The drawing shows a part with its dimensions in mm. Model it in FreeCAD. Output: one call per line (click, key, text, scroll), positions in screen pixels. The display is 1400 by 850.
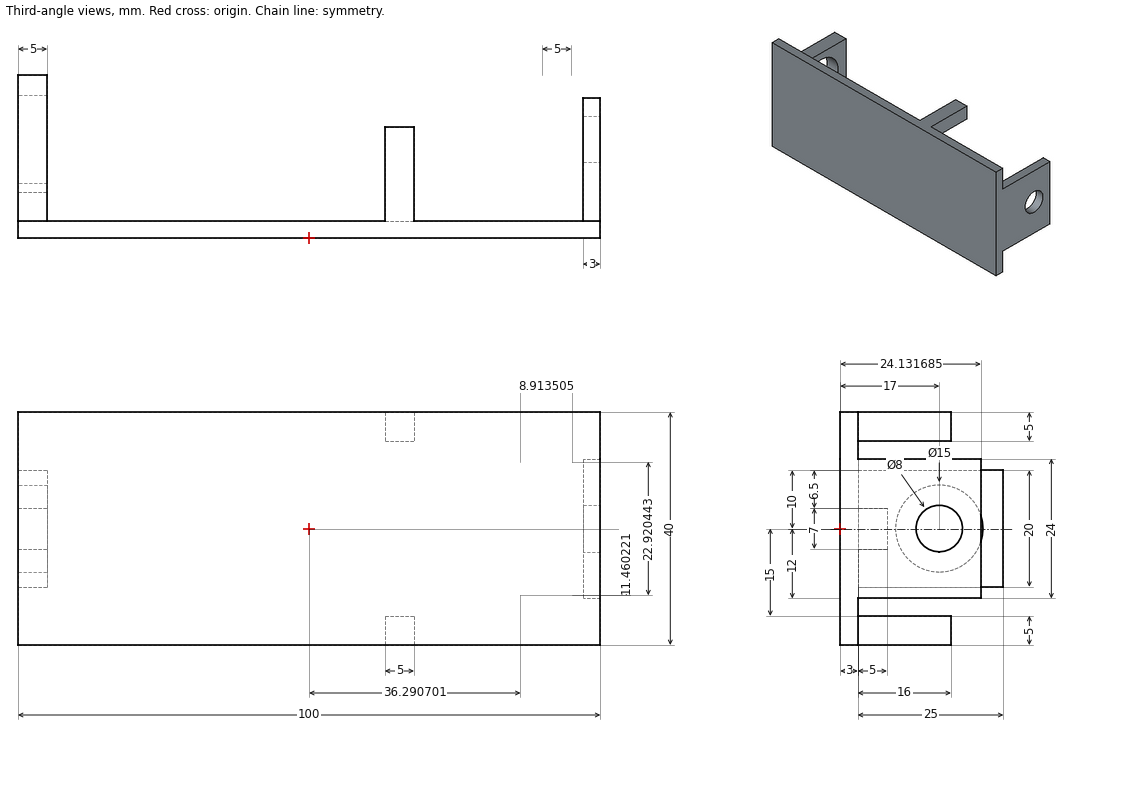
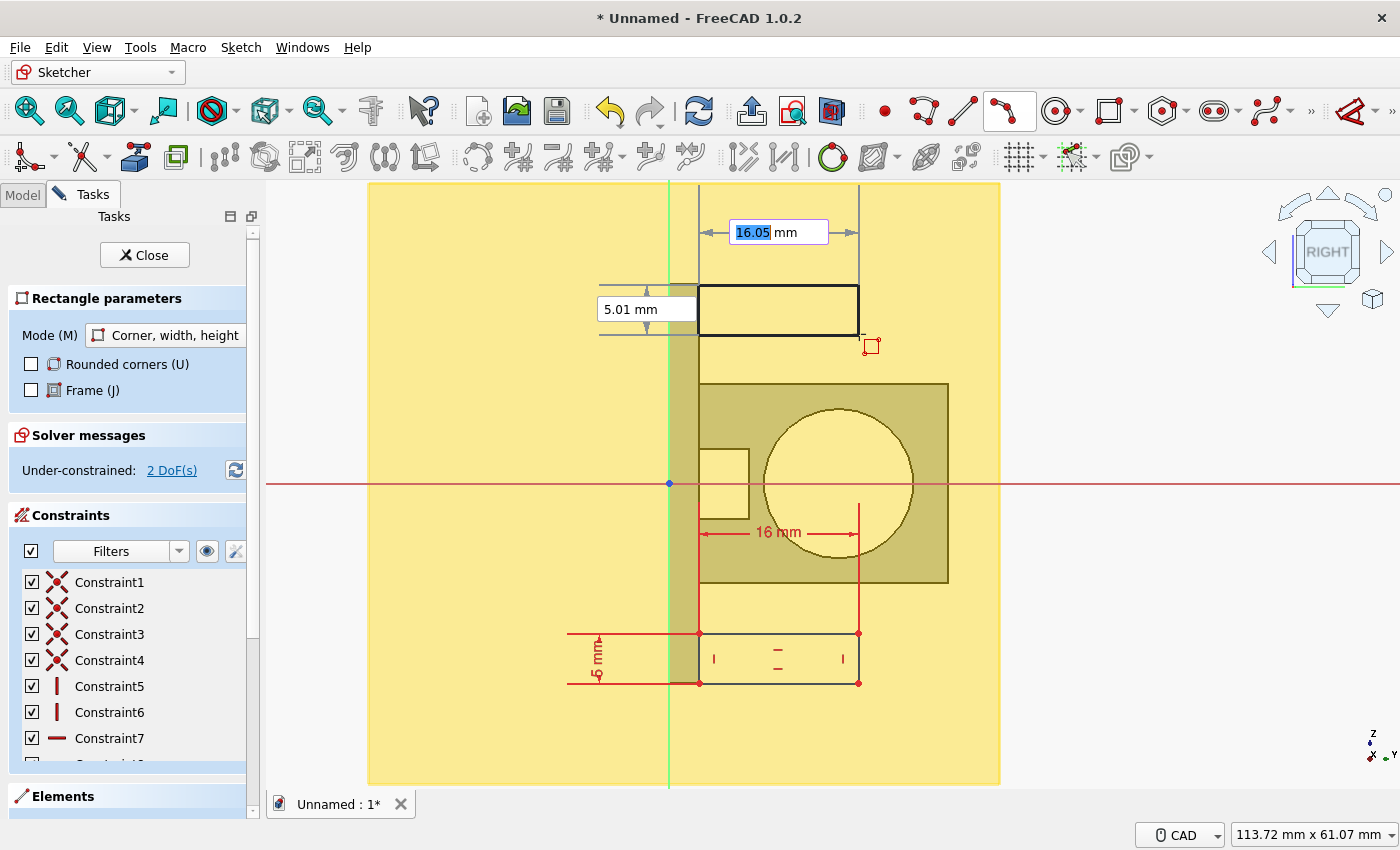
text(16)
key(Tab)
text(5)
key(Return)
key(Escape)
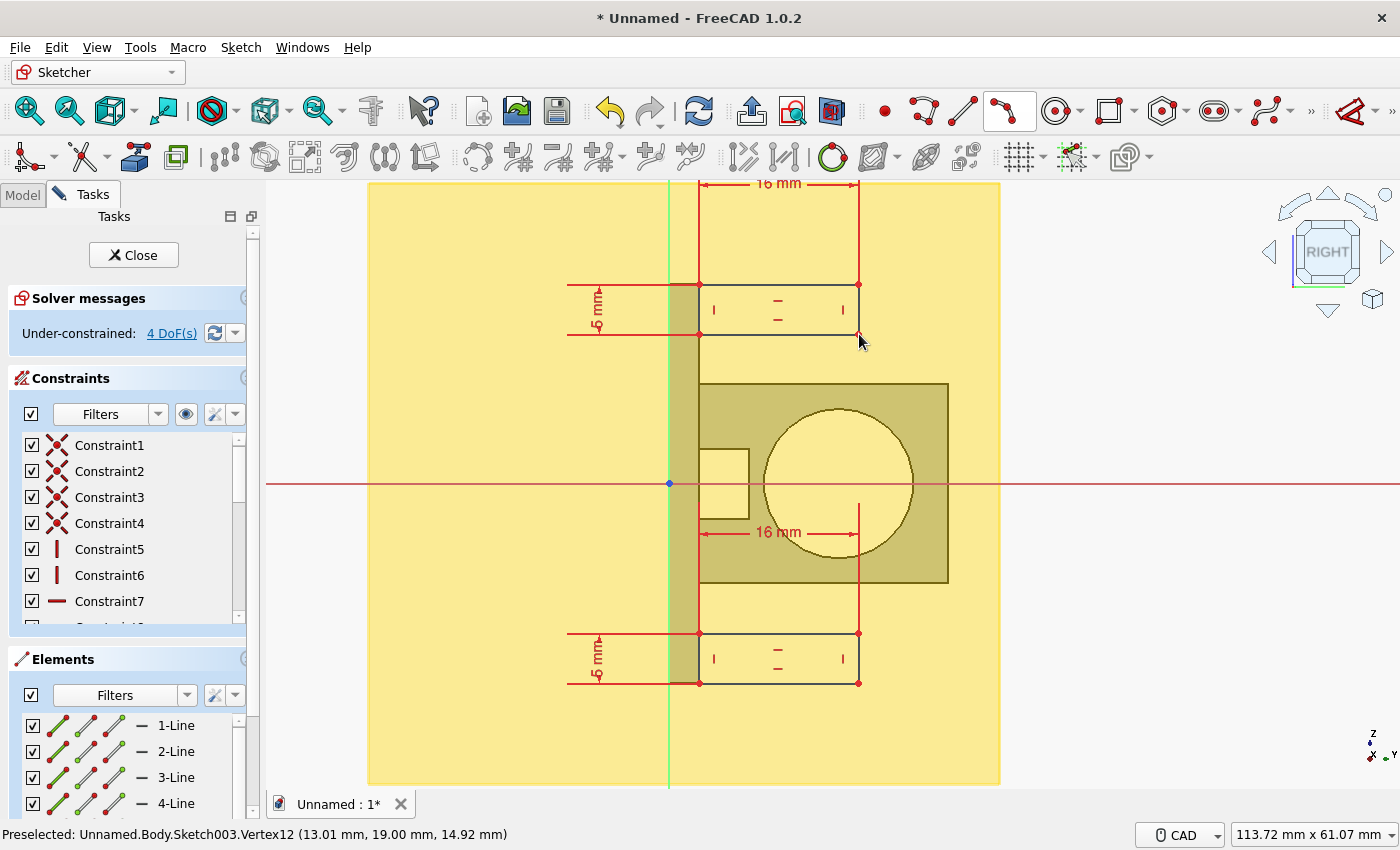
click(699, 684)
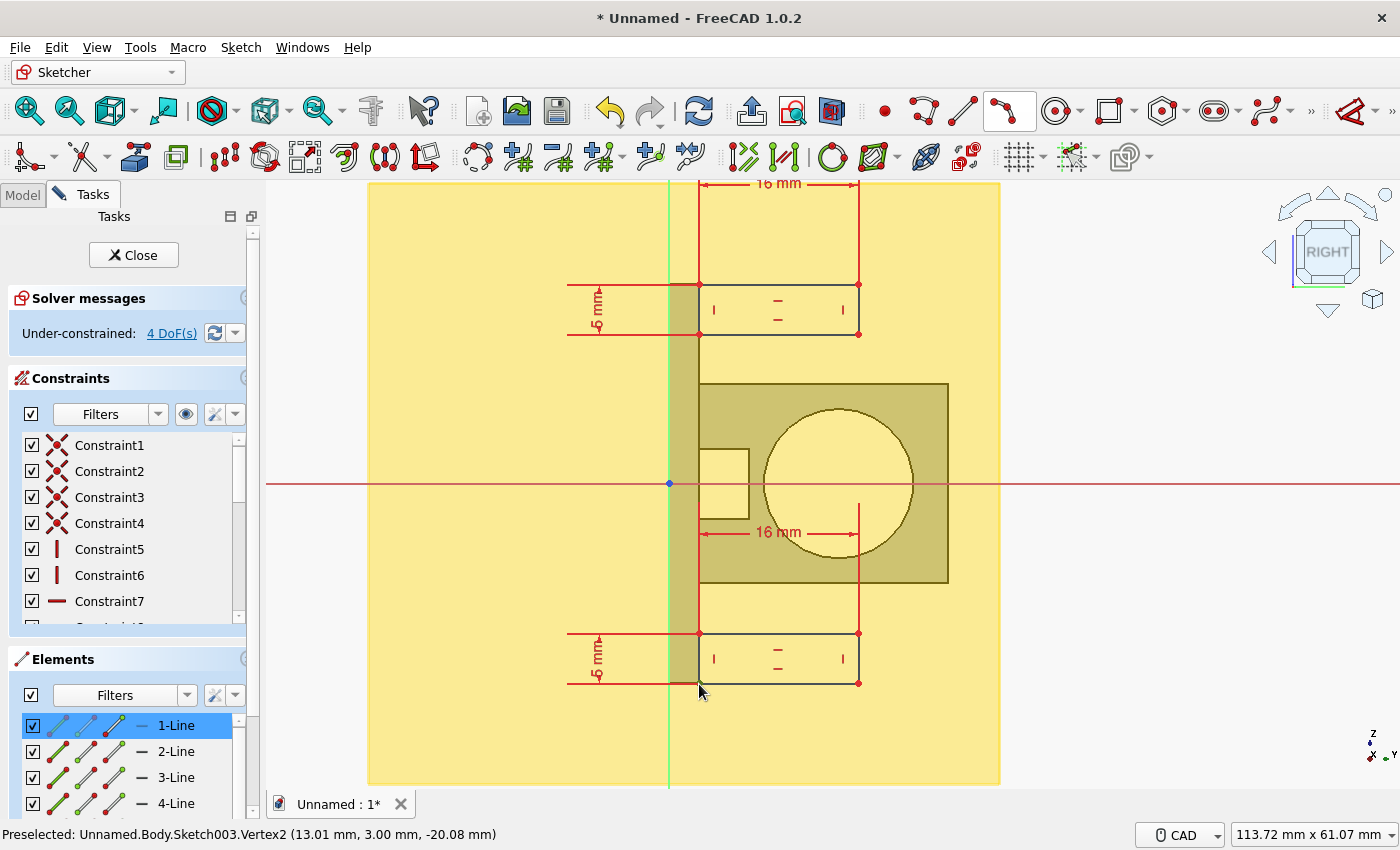
click(699, 285)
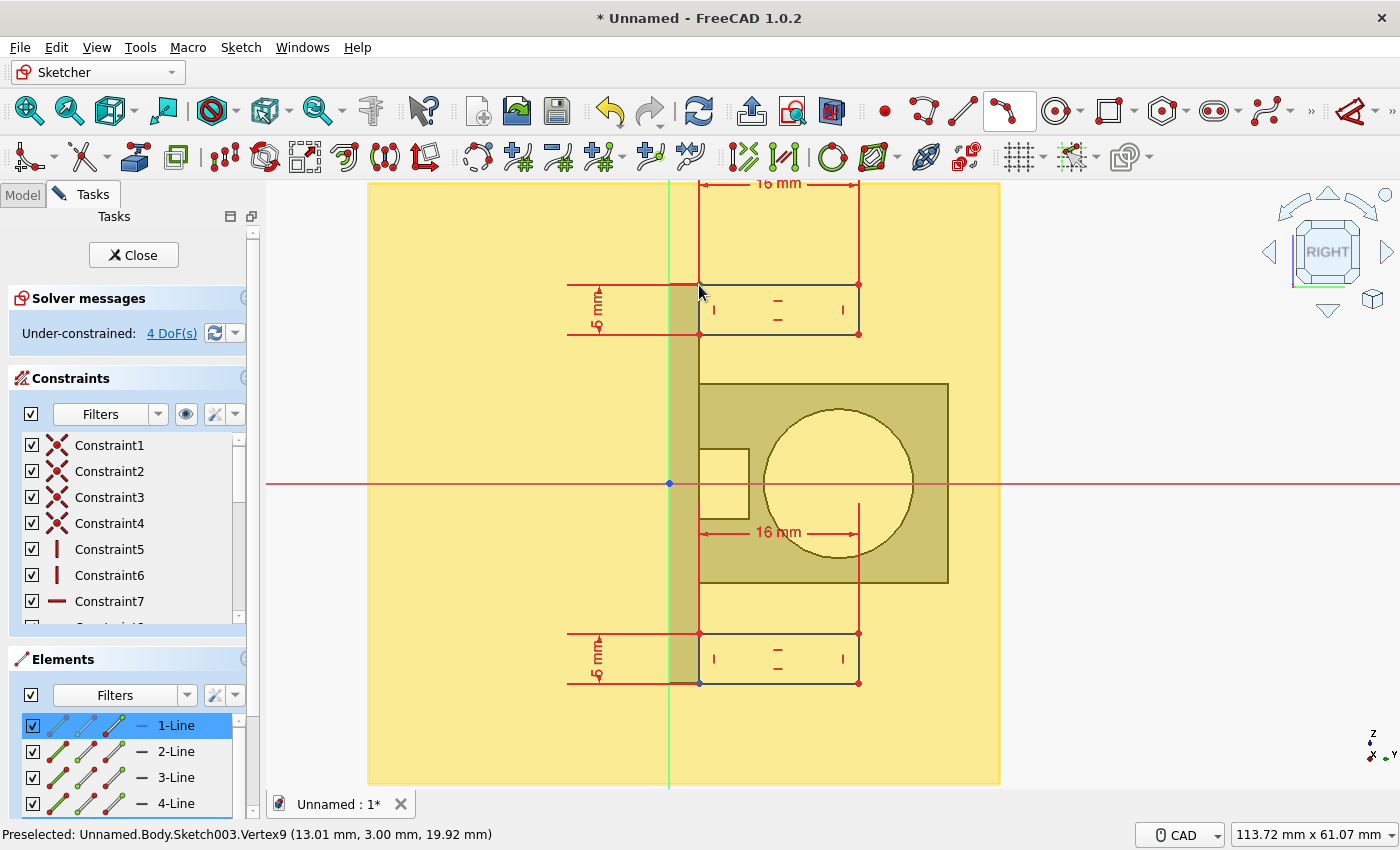
click(361, 484)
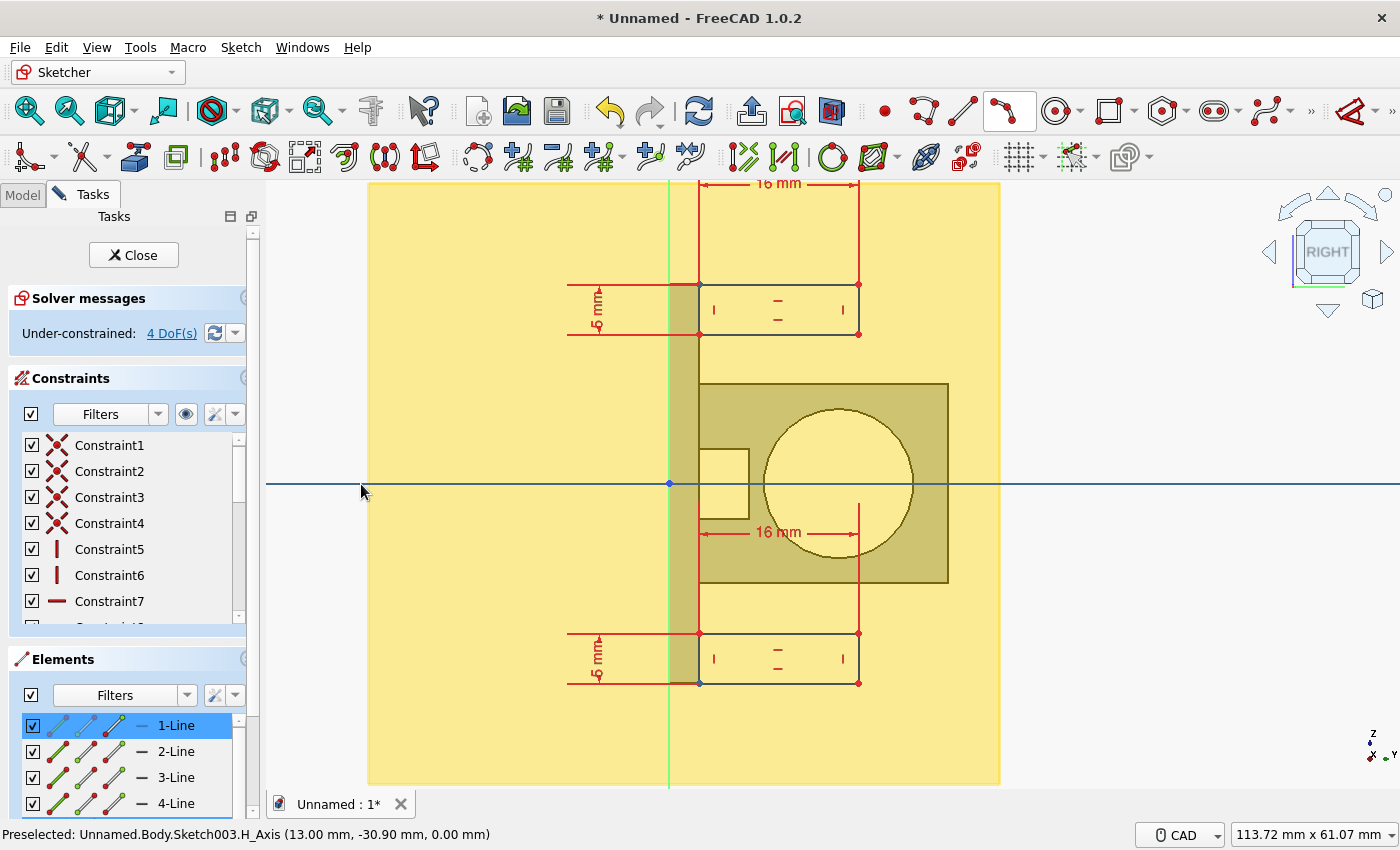
key(s)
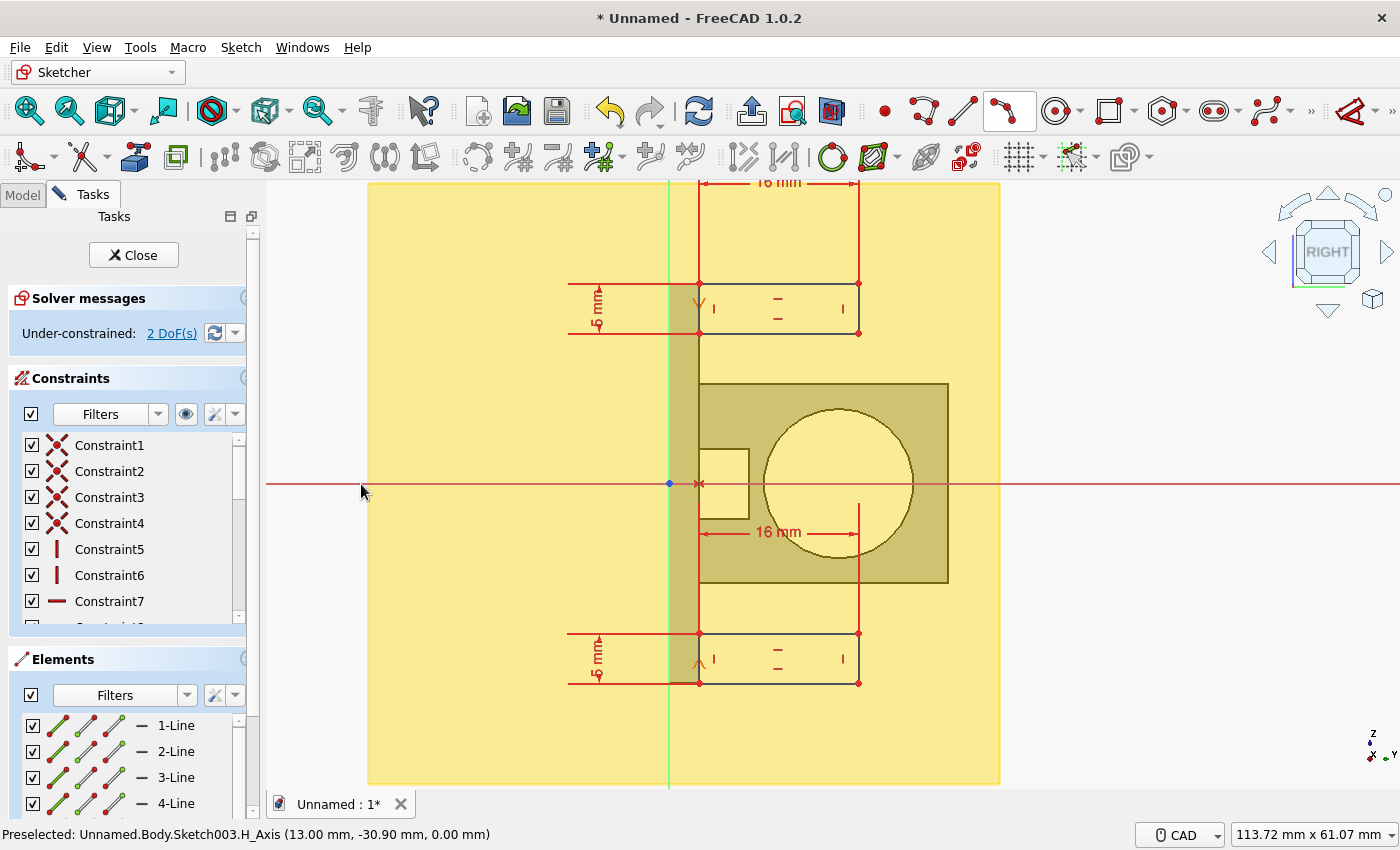
click(1350, 112)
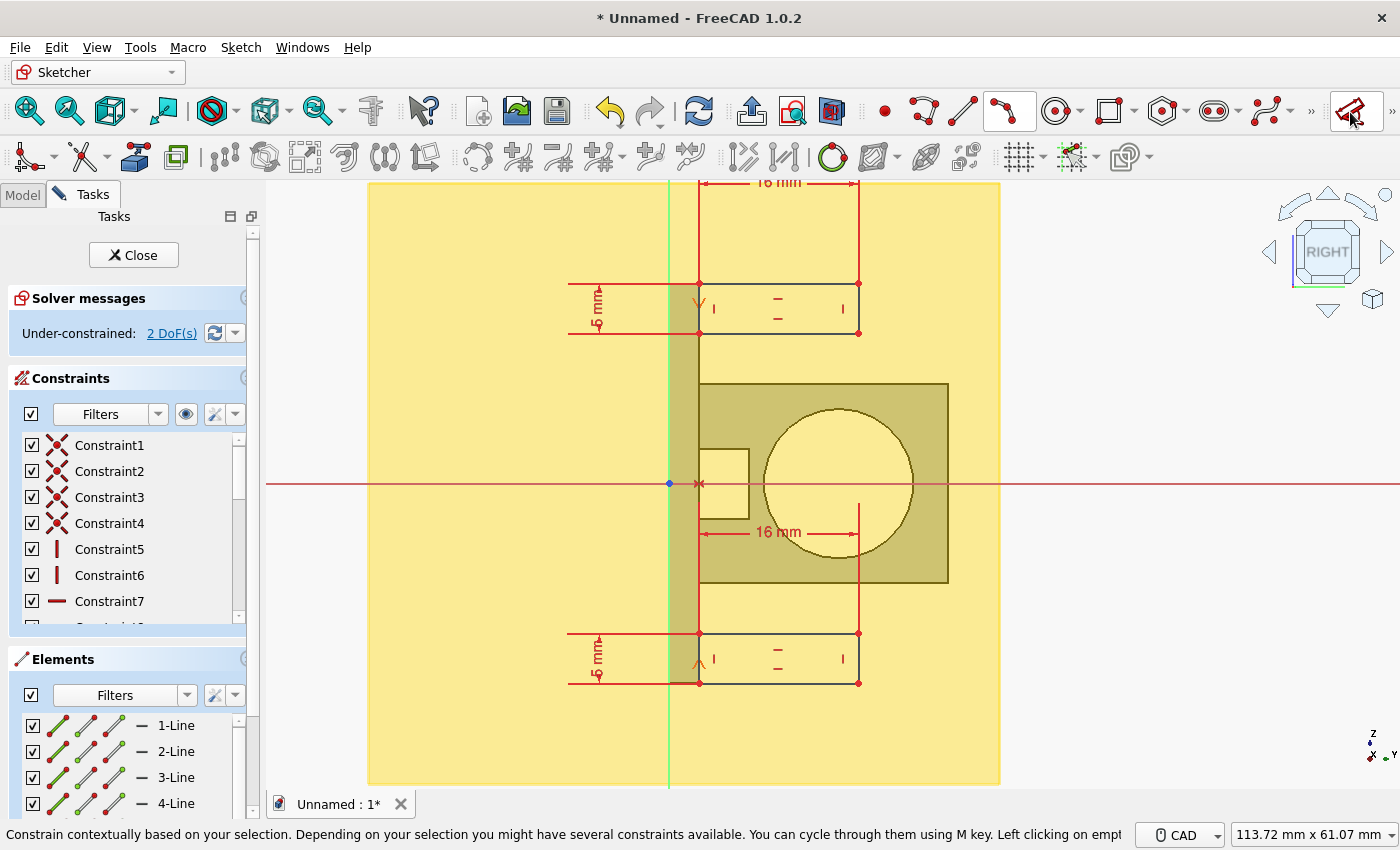
scroll(699, 634, up, 2)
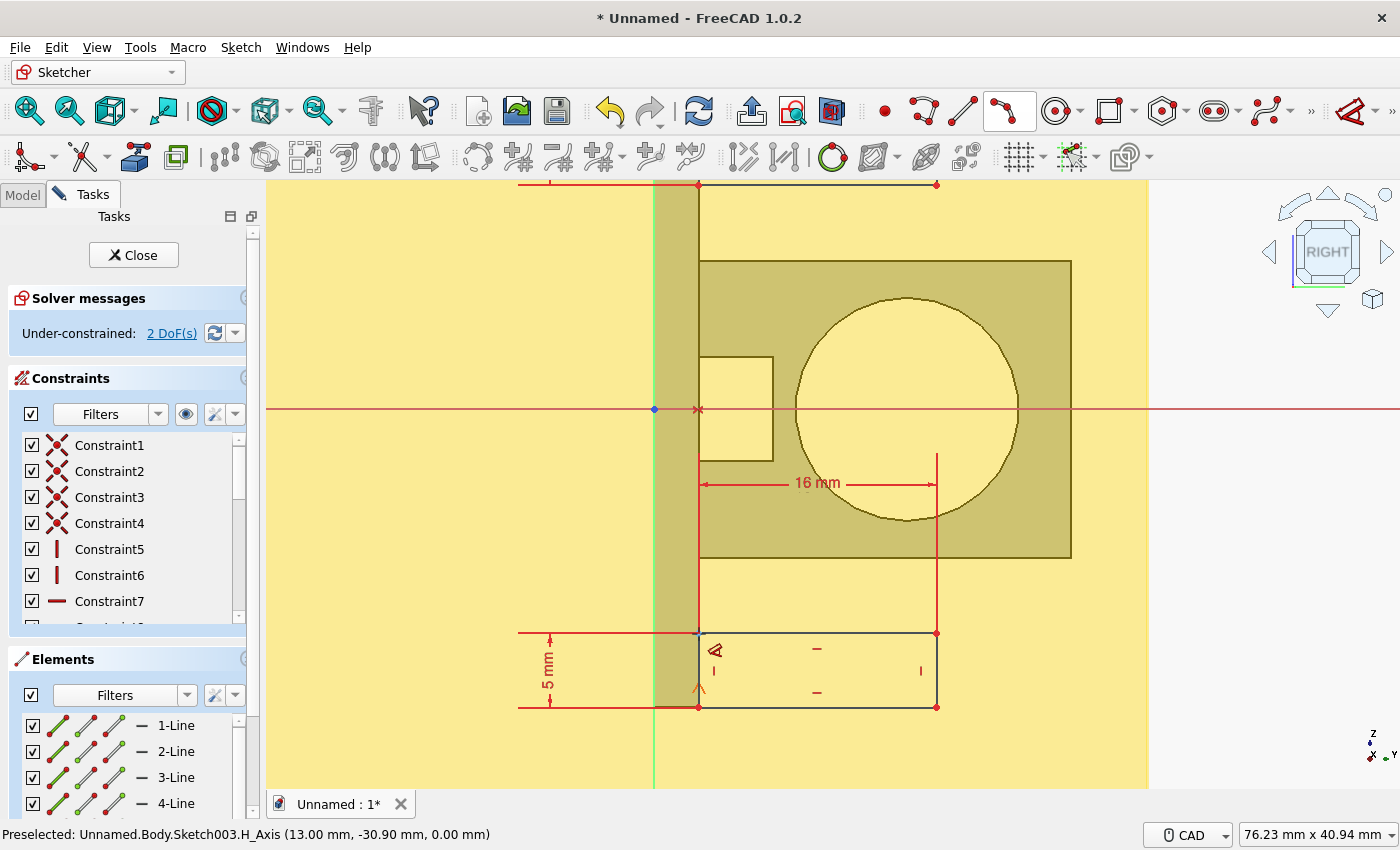
click(699, 633)
click(677, 667)